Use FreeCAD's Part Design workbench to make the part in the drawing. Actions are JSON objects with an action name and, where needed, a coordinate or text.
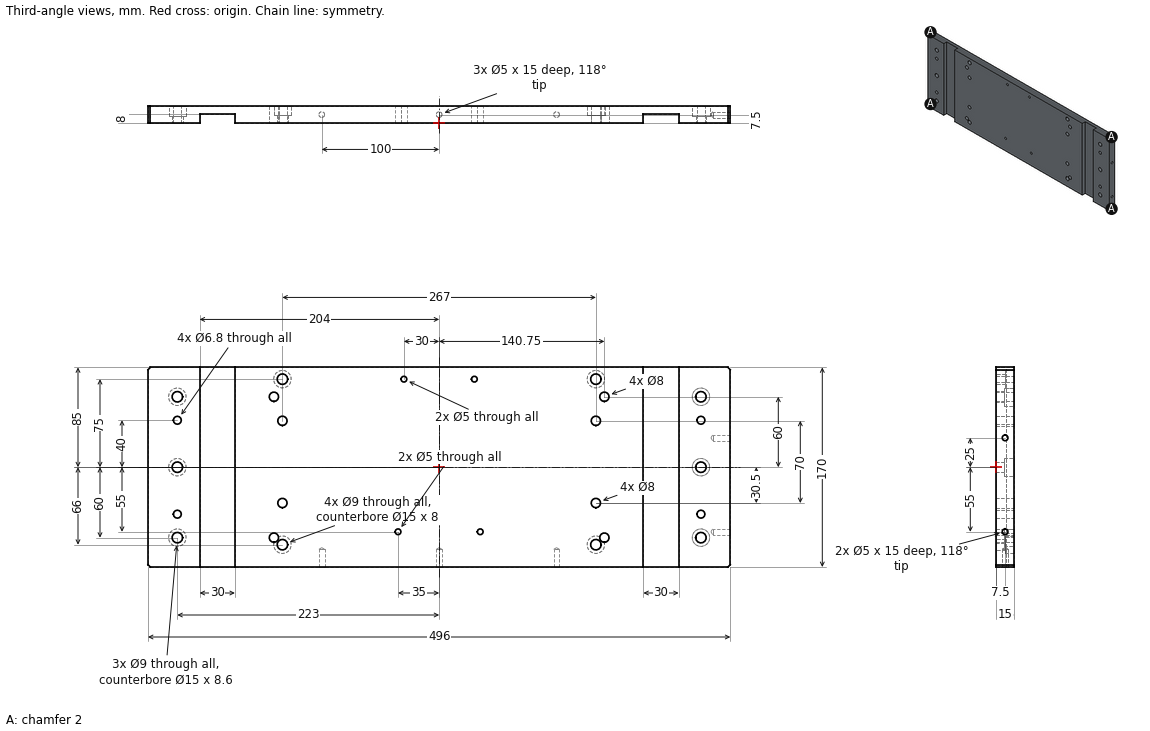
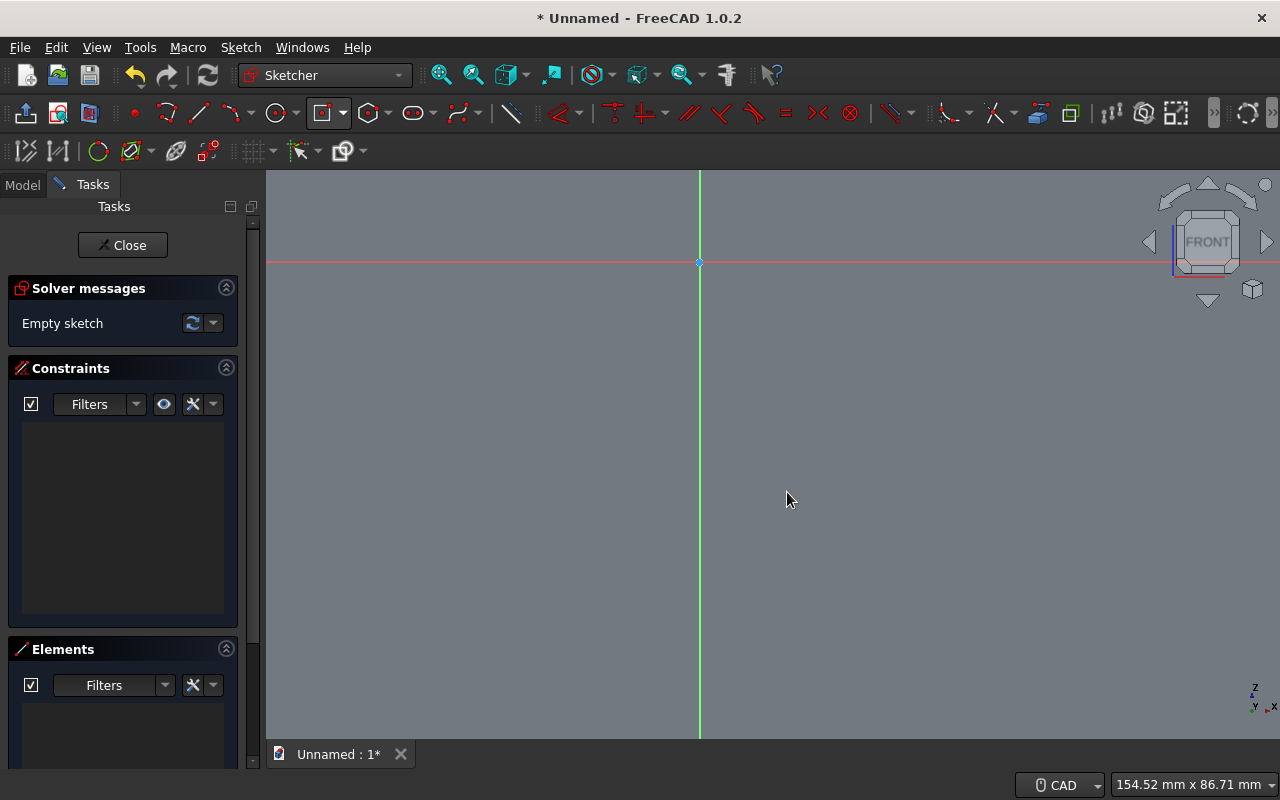
{"action": "left_click", "coordinate": [276, 114]}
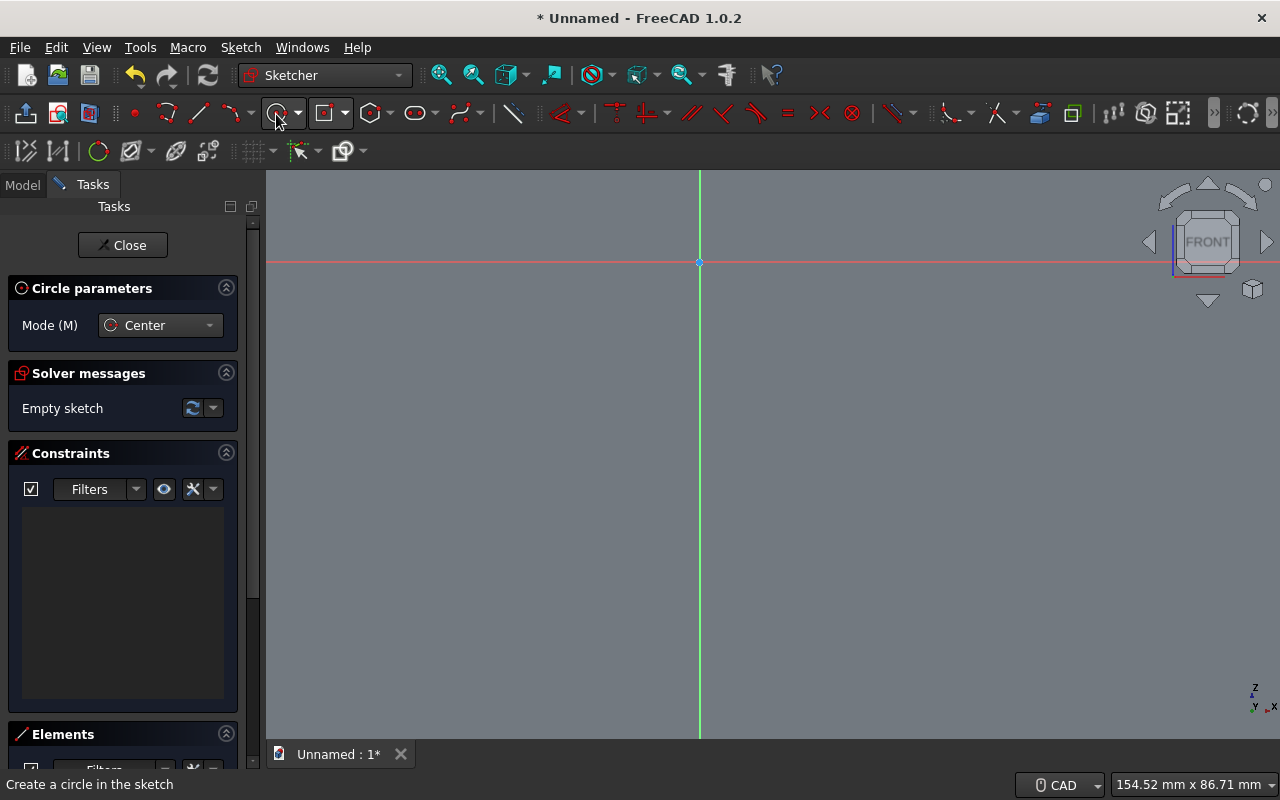
{"action": "scroll", "coordinate": [470, 623], "scroll_direction": "up", "scroll_amount": 2}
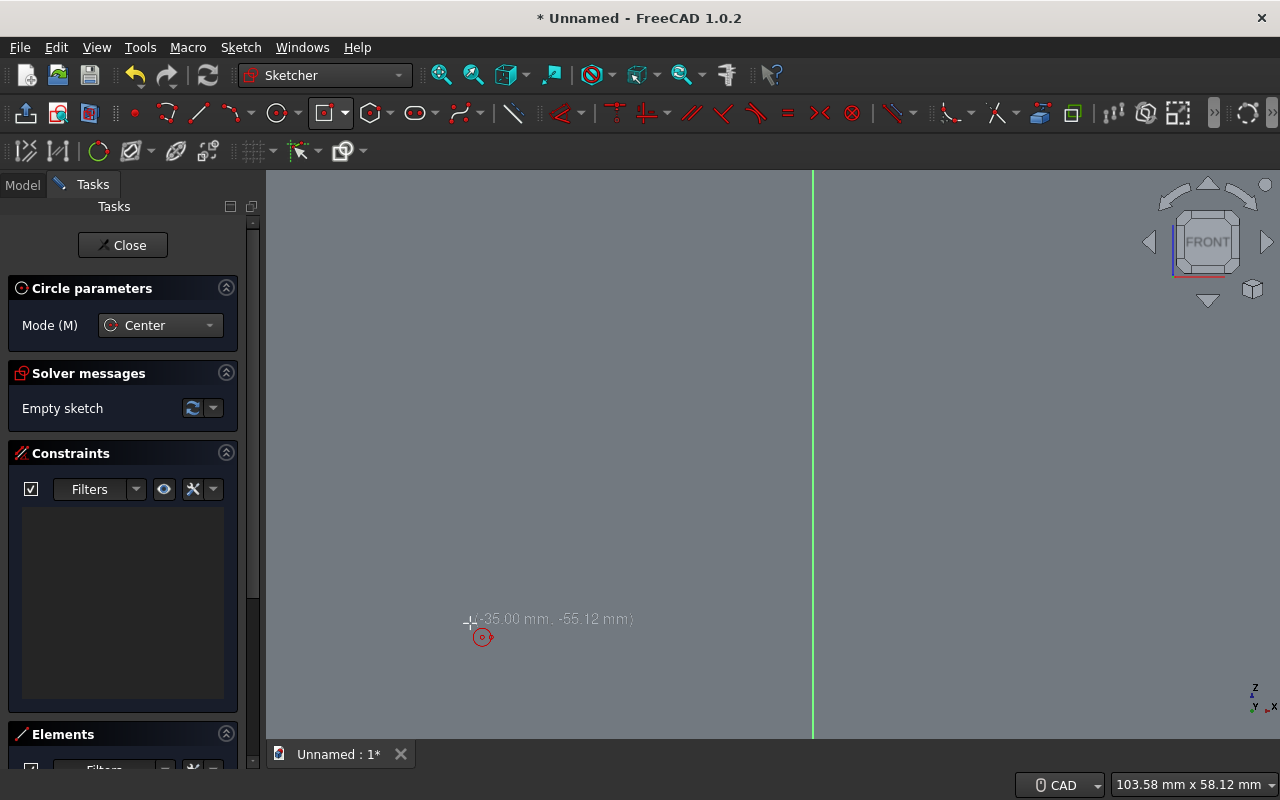
{"action": "left_click", "coordinate": [470, 623]}
{"action": "mouse_move", "coordinate": [487, 606]}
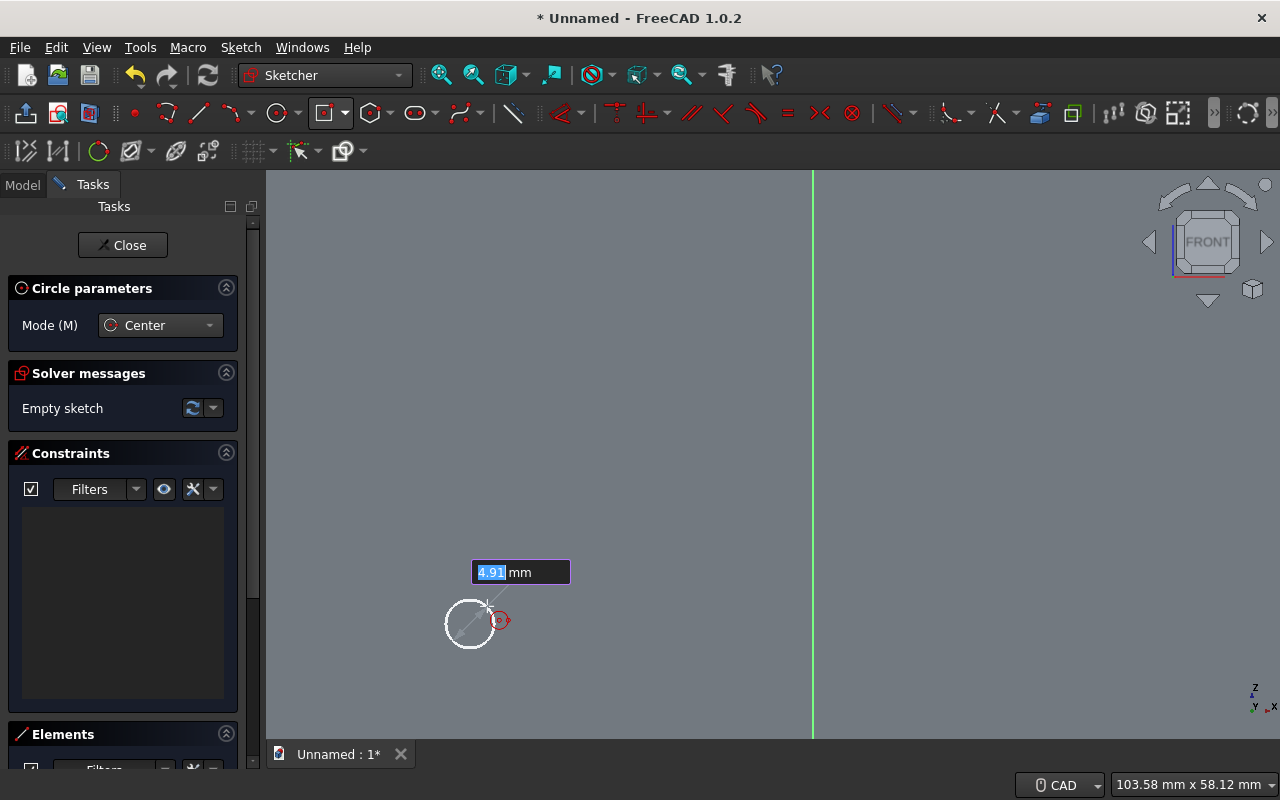
{"action": "type", "text": "5"}
{"action": "key", "text": "Return"}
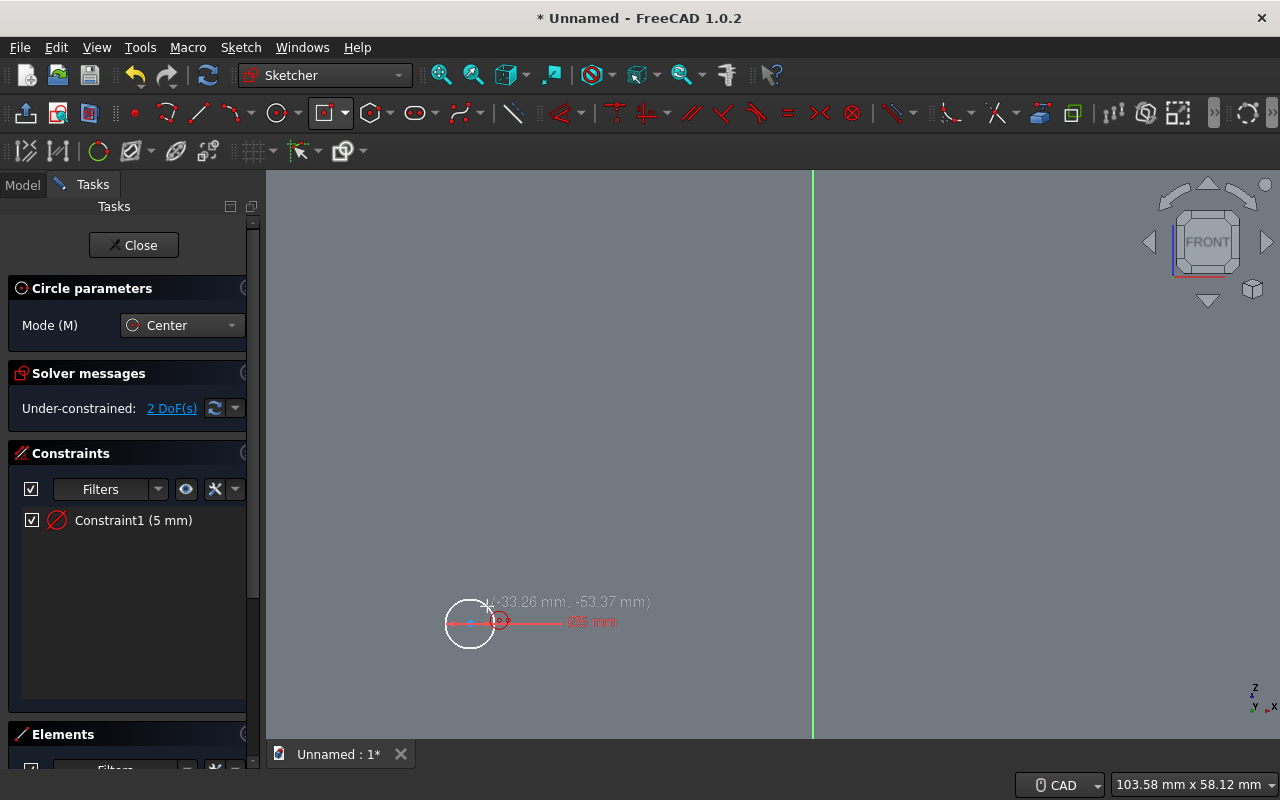
{"action": "scroll", "coordinate": [485, 635], "scroll_direction": "down", "scroll_amount": 2}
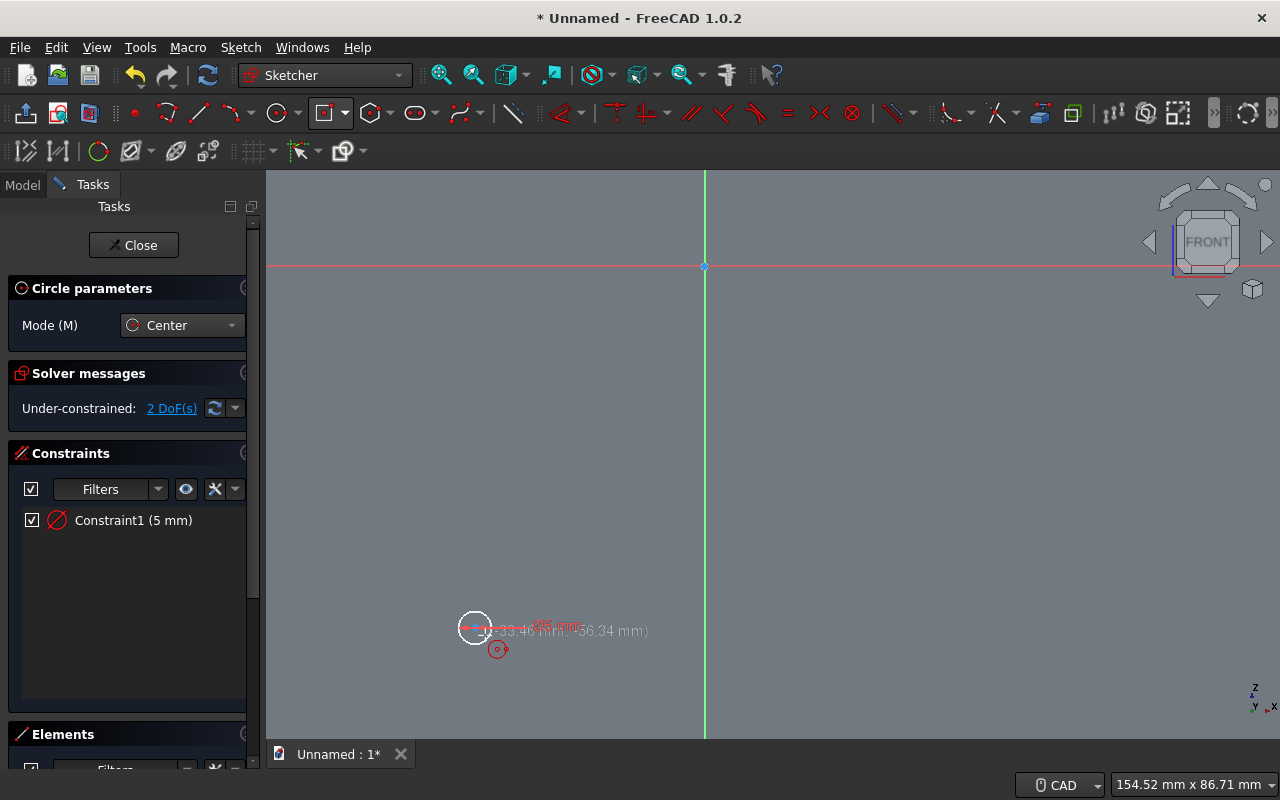
{"action": "scroll", "coordinate": [934, 627], "scroll_direction": "up", "scroll_amount": 2}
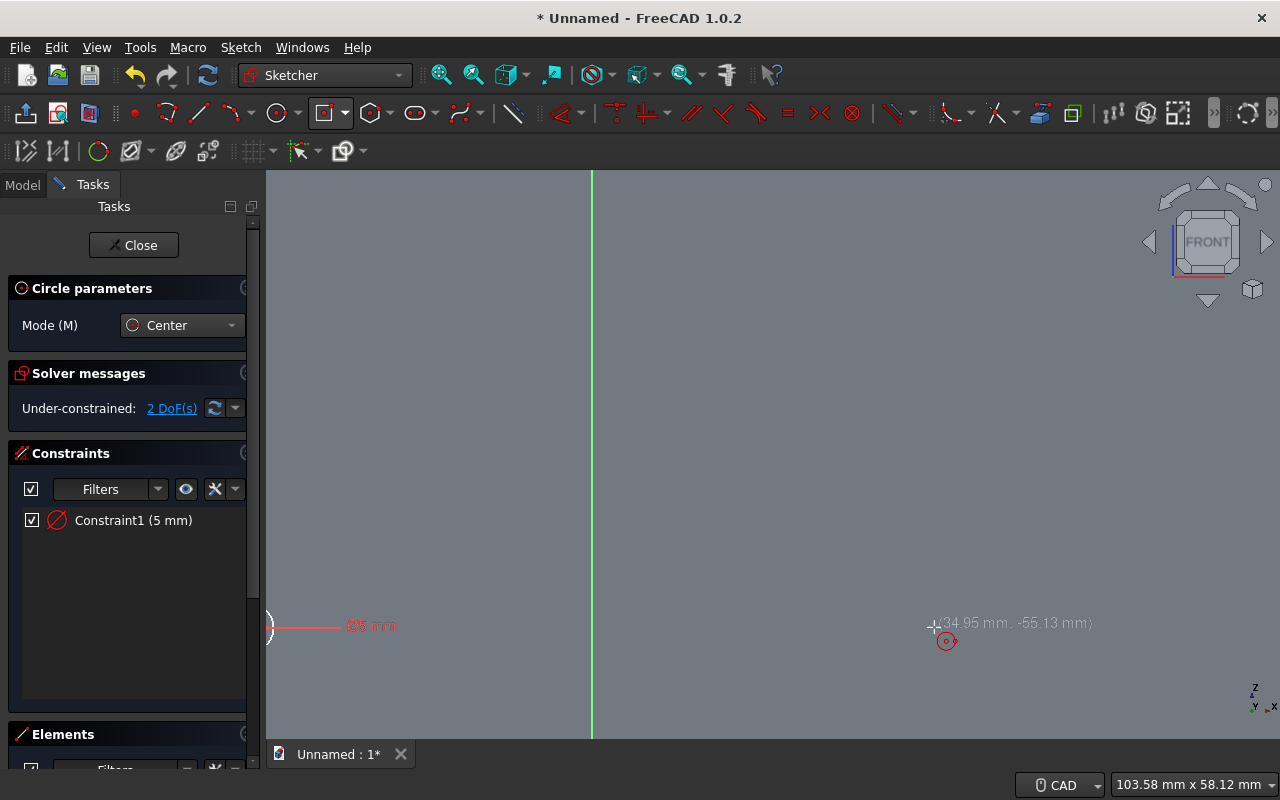
{"action": "left_click", "coordinate": [934, 627]}
{"action": "mouse_move", "coordinate": [951, 610]}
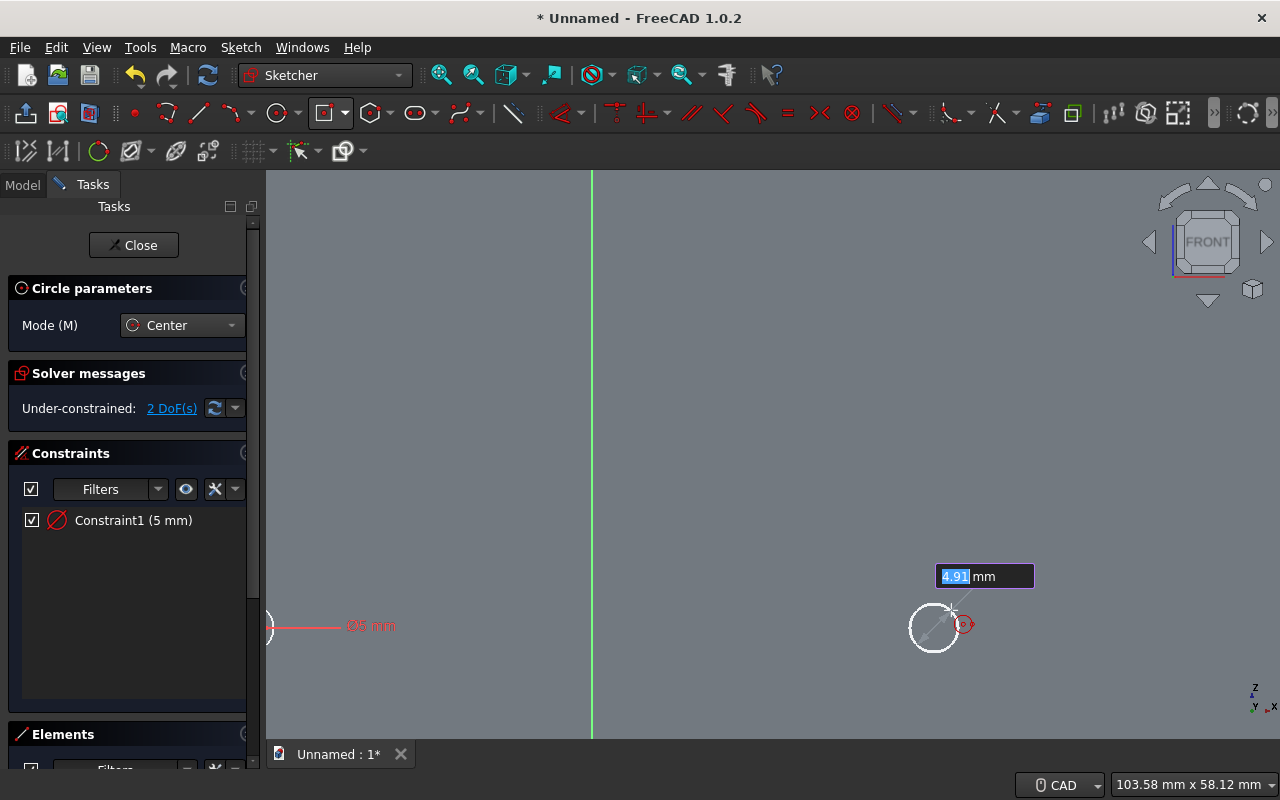
{"action": "type", "text": "5"}
{"action": "key", "text": "Return"}
{"action": "key", "text": "Escape"}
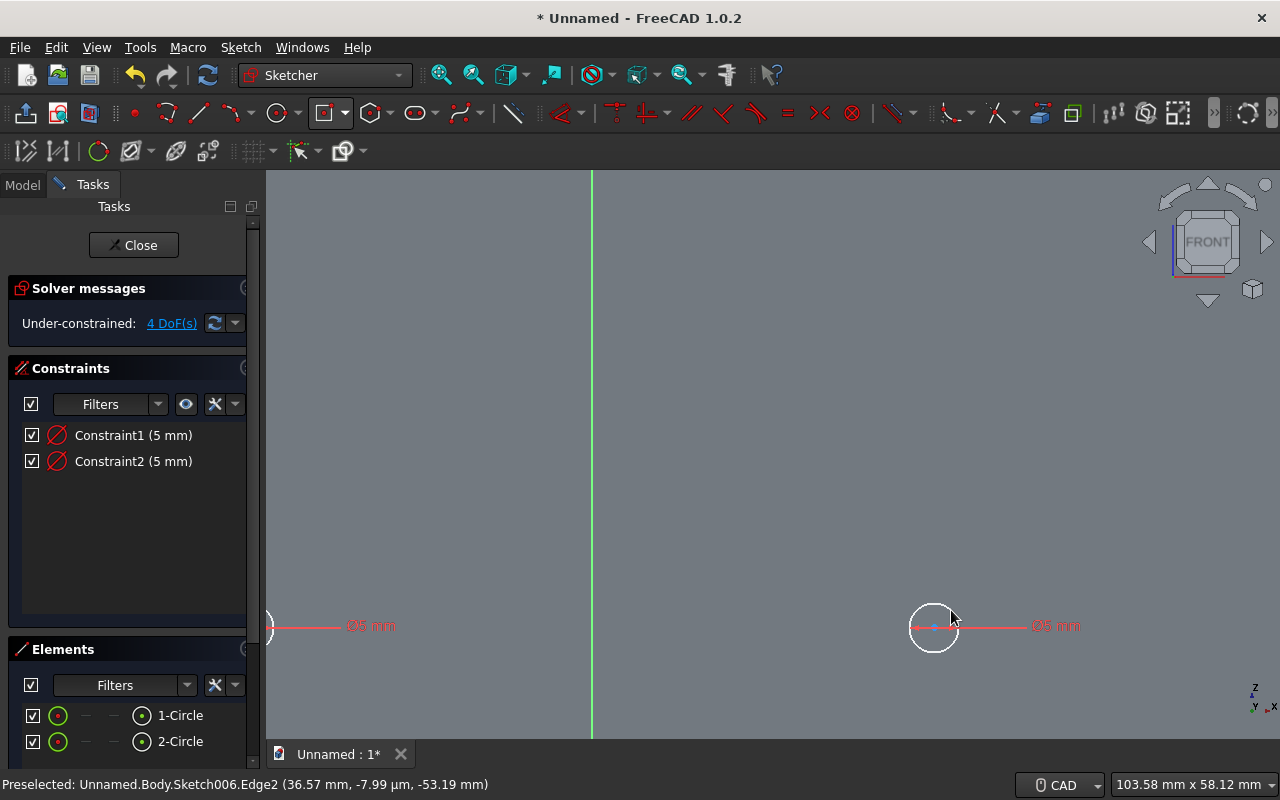
{"action": "scroll", "coordinate": [934, 627], "scroll_direction": "down", "scroll_amount": 2}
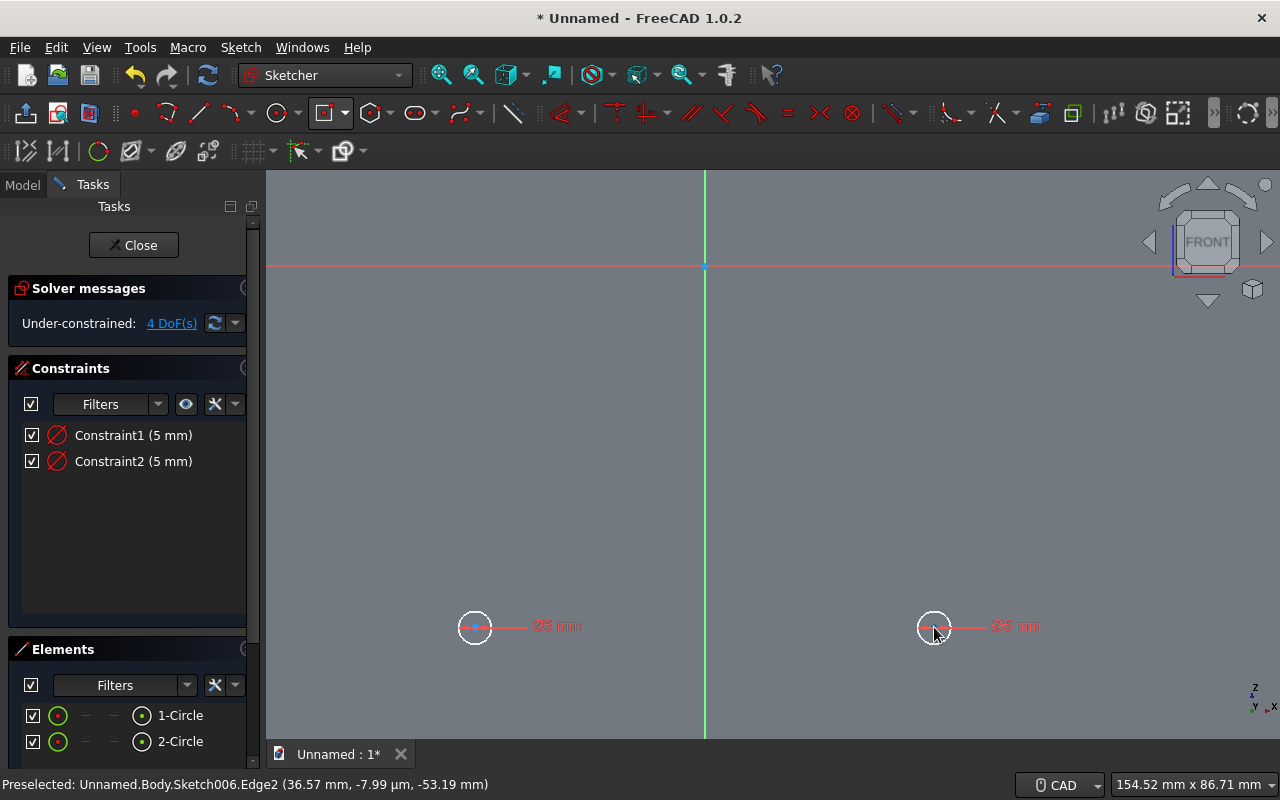
{"action": "left_click", "coordinate": [475, 628]}